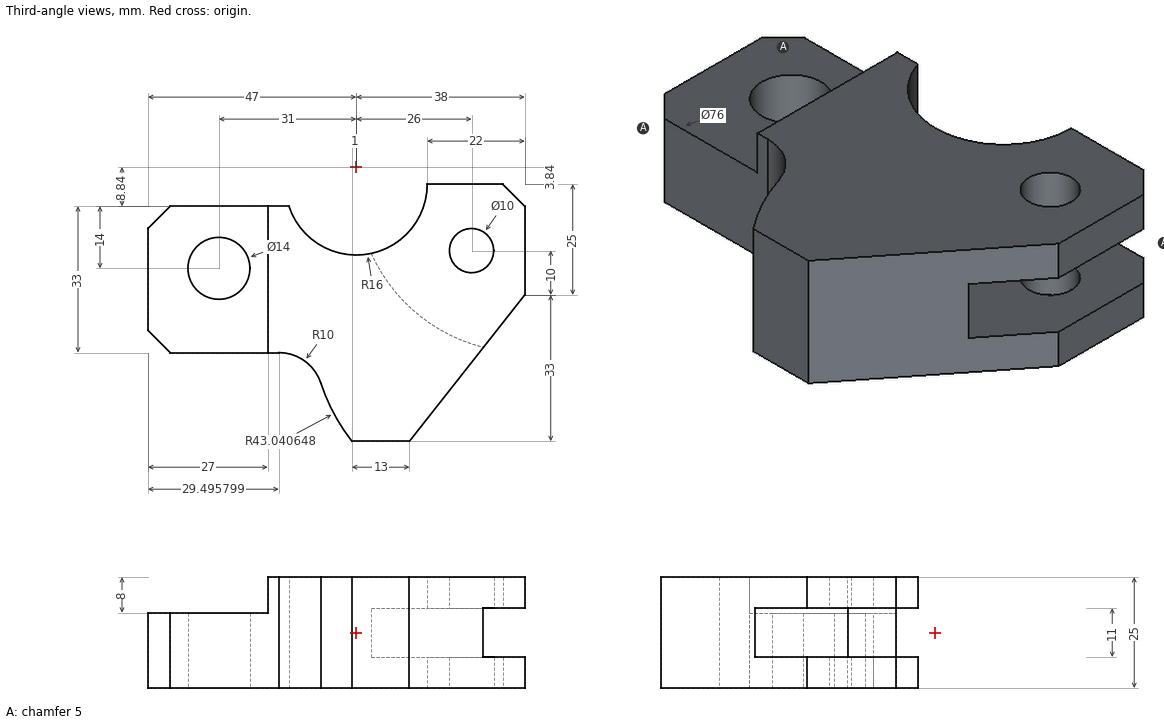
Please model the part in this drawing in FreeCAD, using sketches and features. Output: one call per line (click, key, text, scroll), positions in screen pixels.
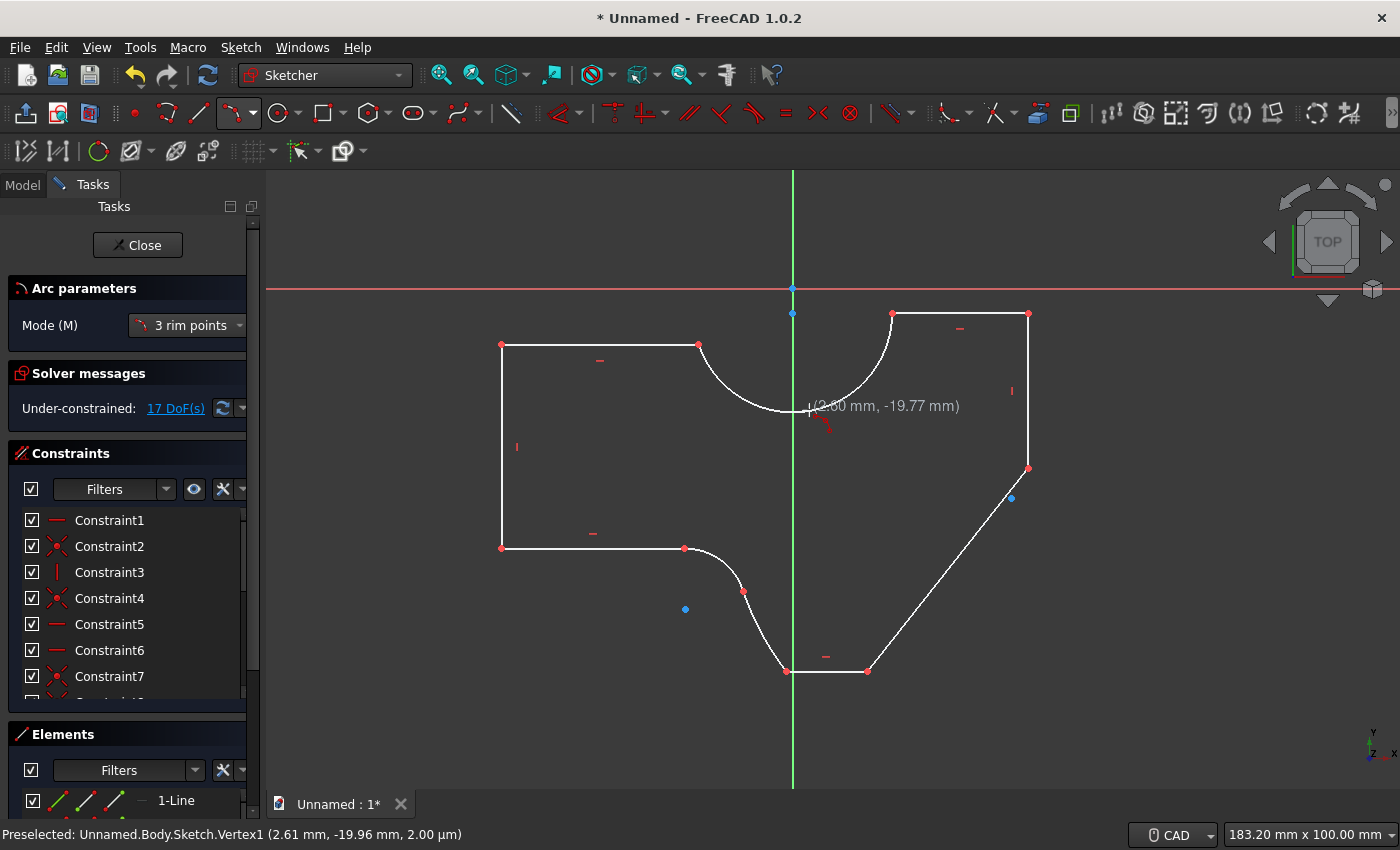
key(g)
key(c)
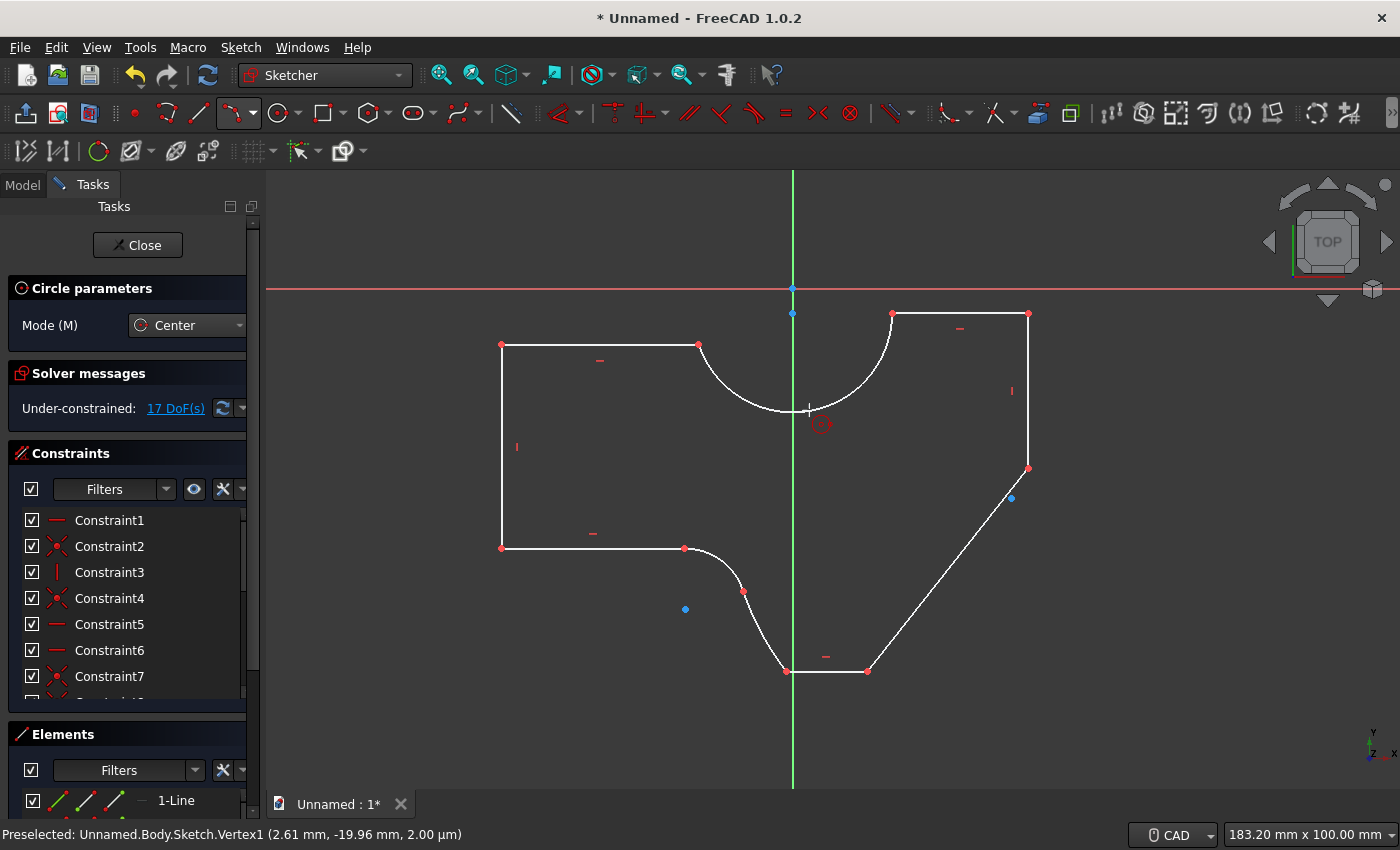
click(601, 430)
move(632, 399)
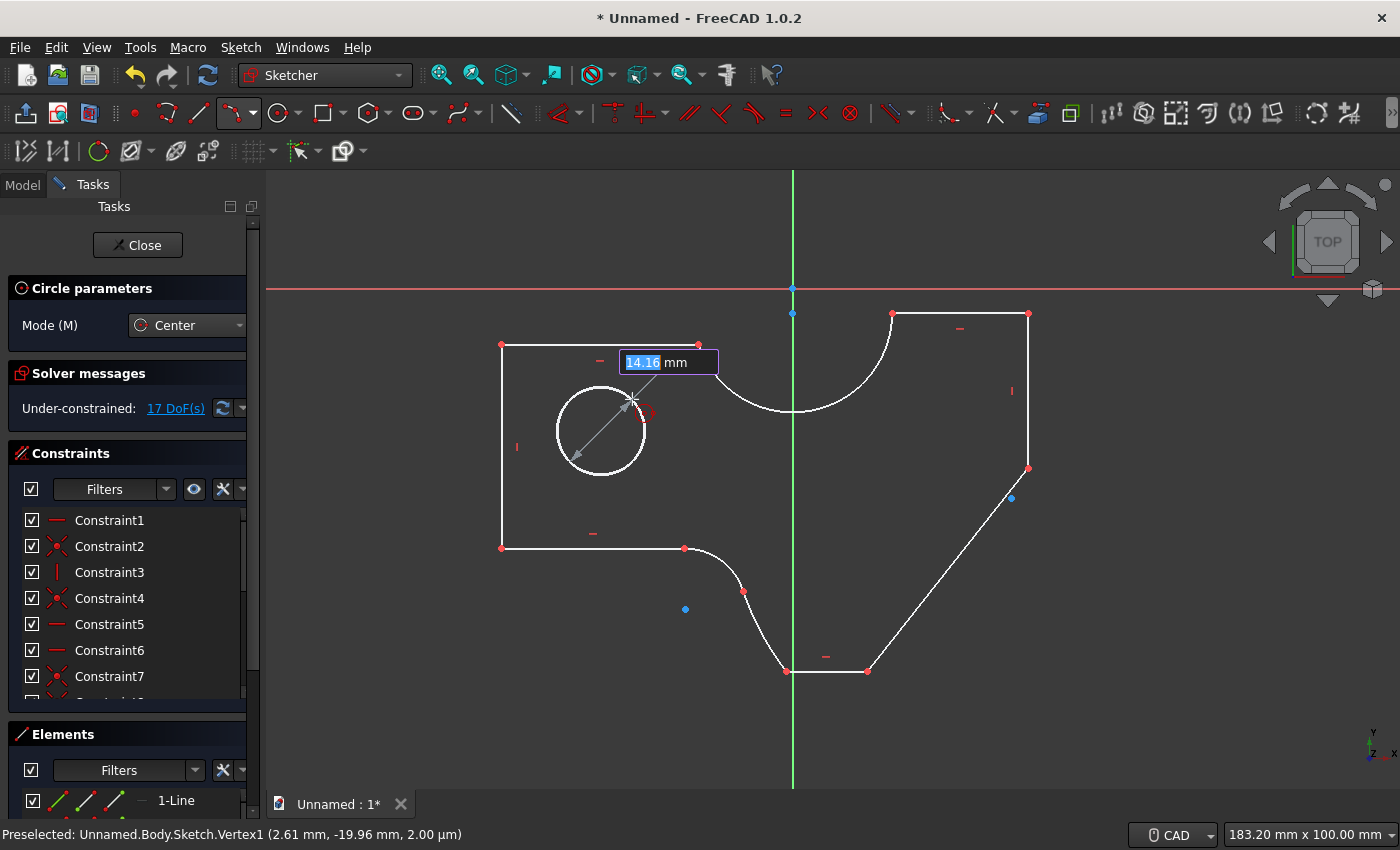
text(14)
key(Return)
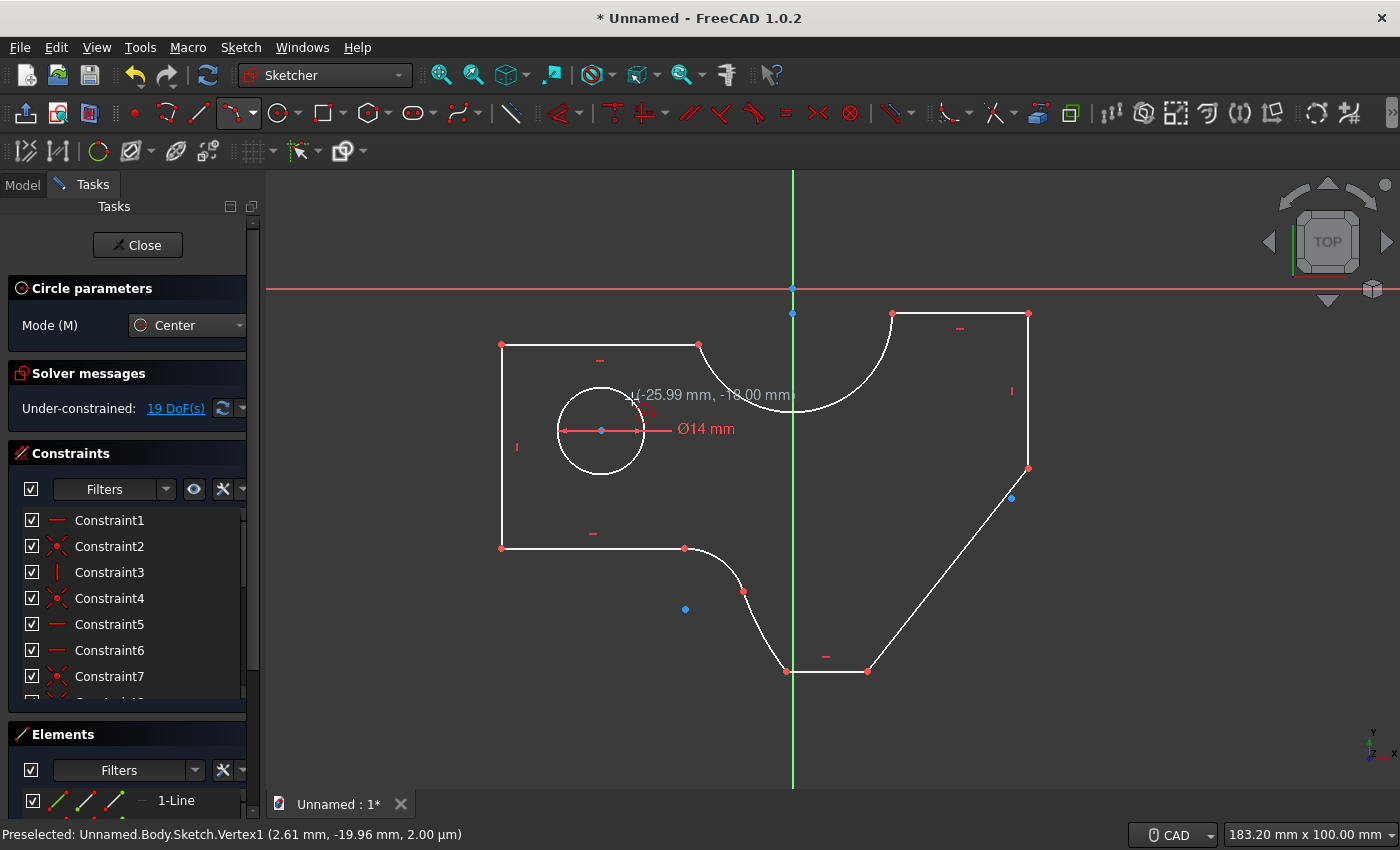
click(954, 405)
move(976, 383)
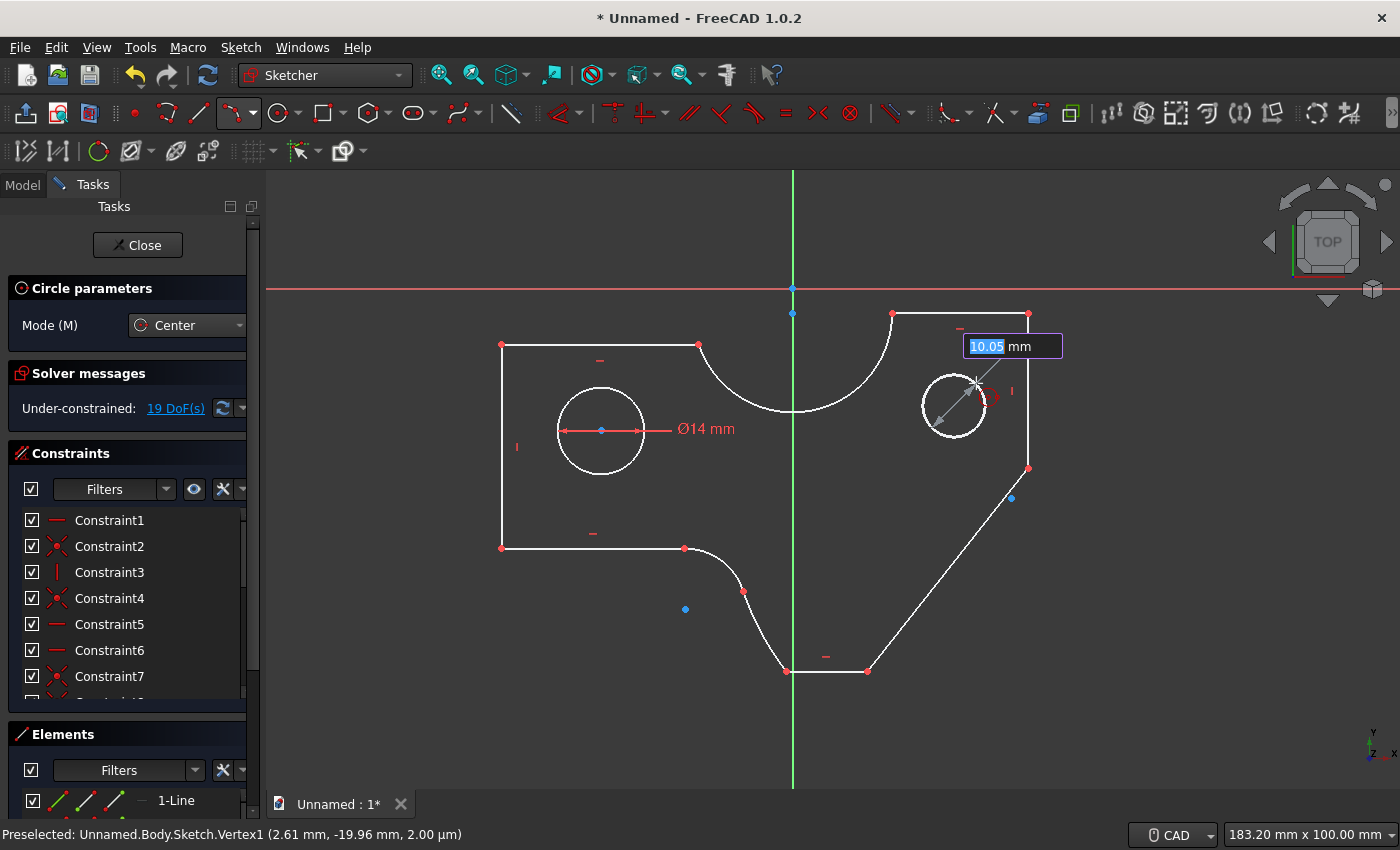
text(10)
key(Return)
key(Escape)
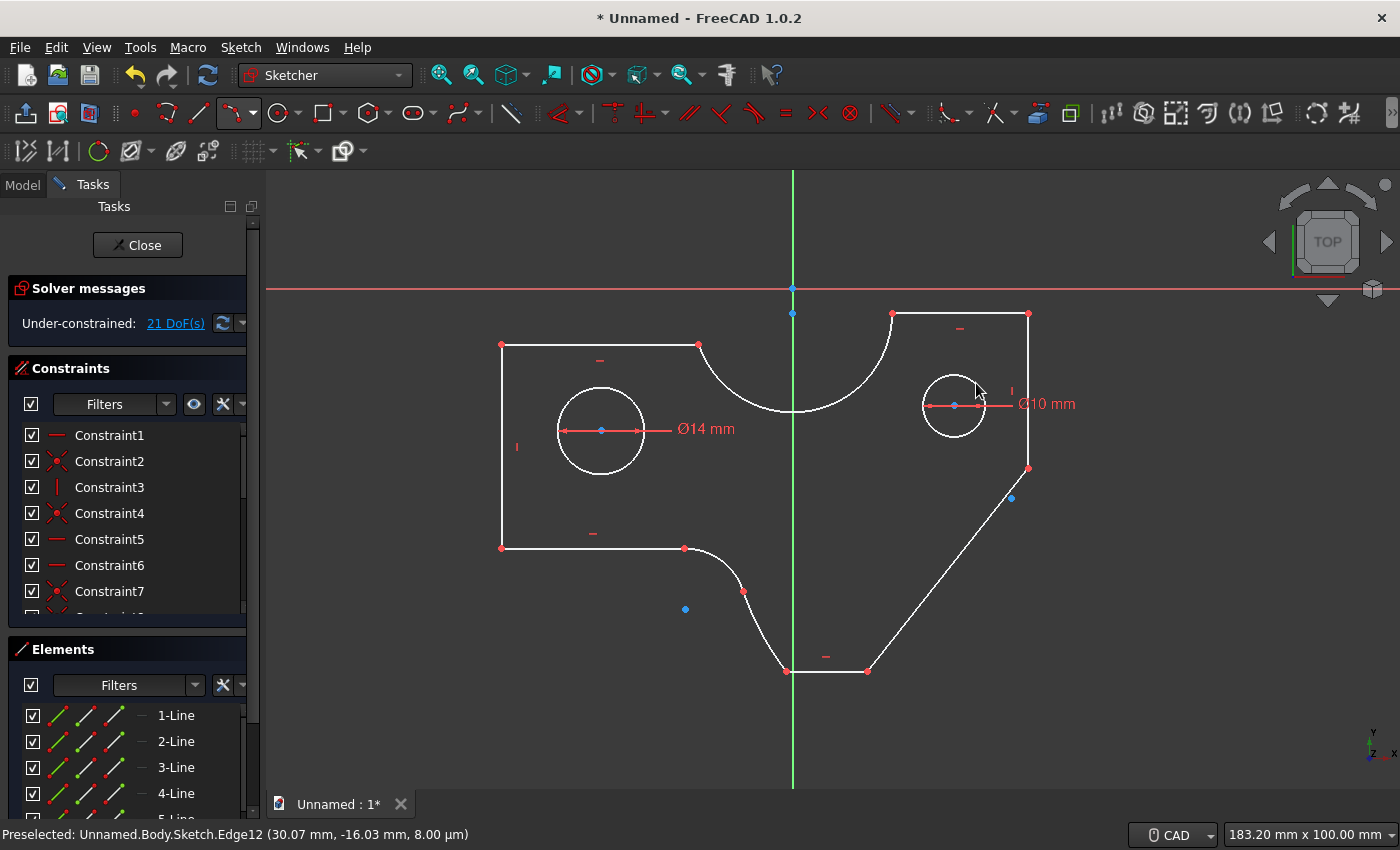
click(557, 549)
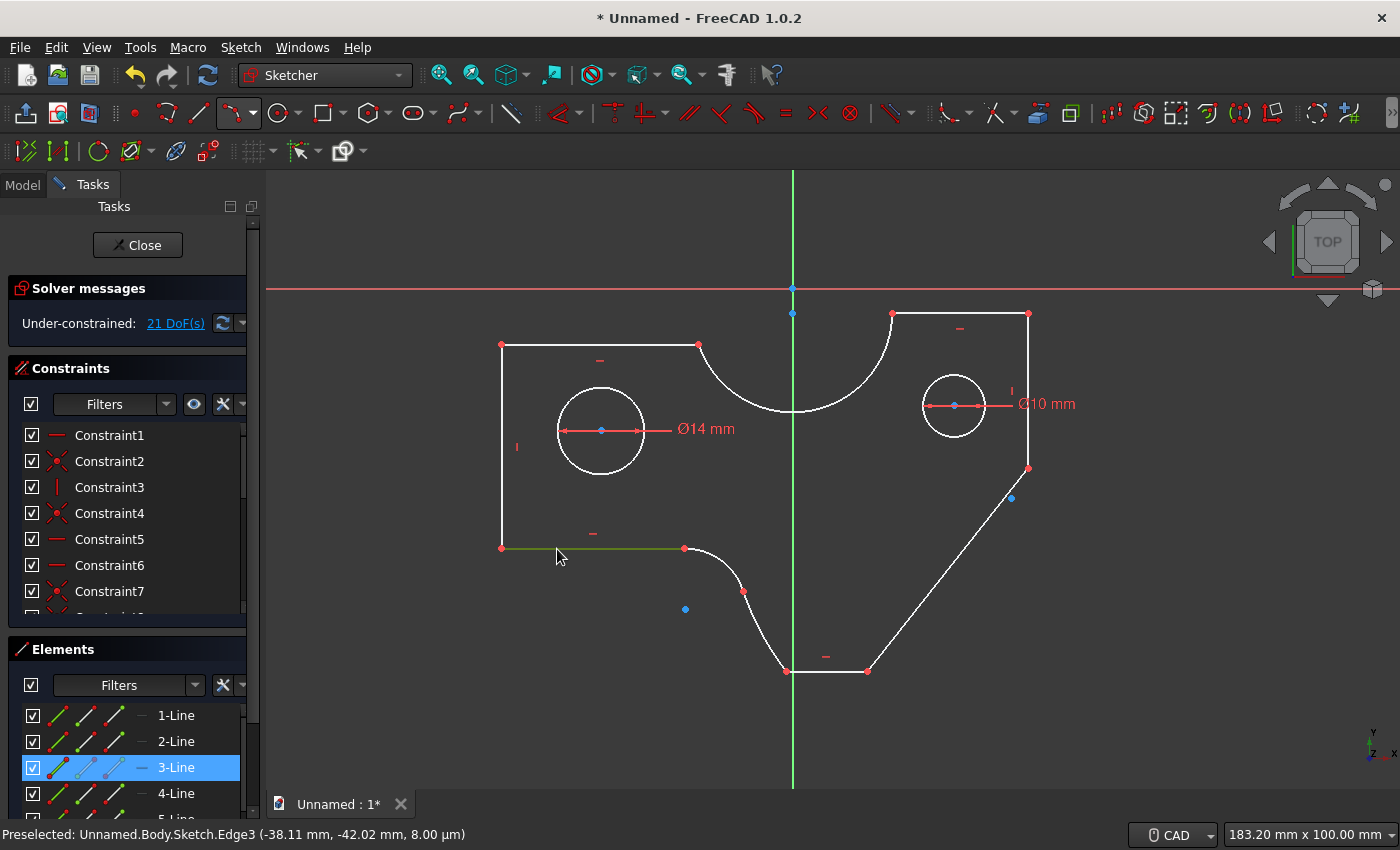
click(732, 571)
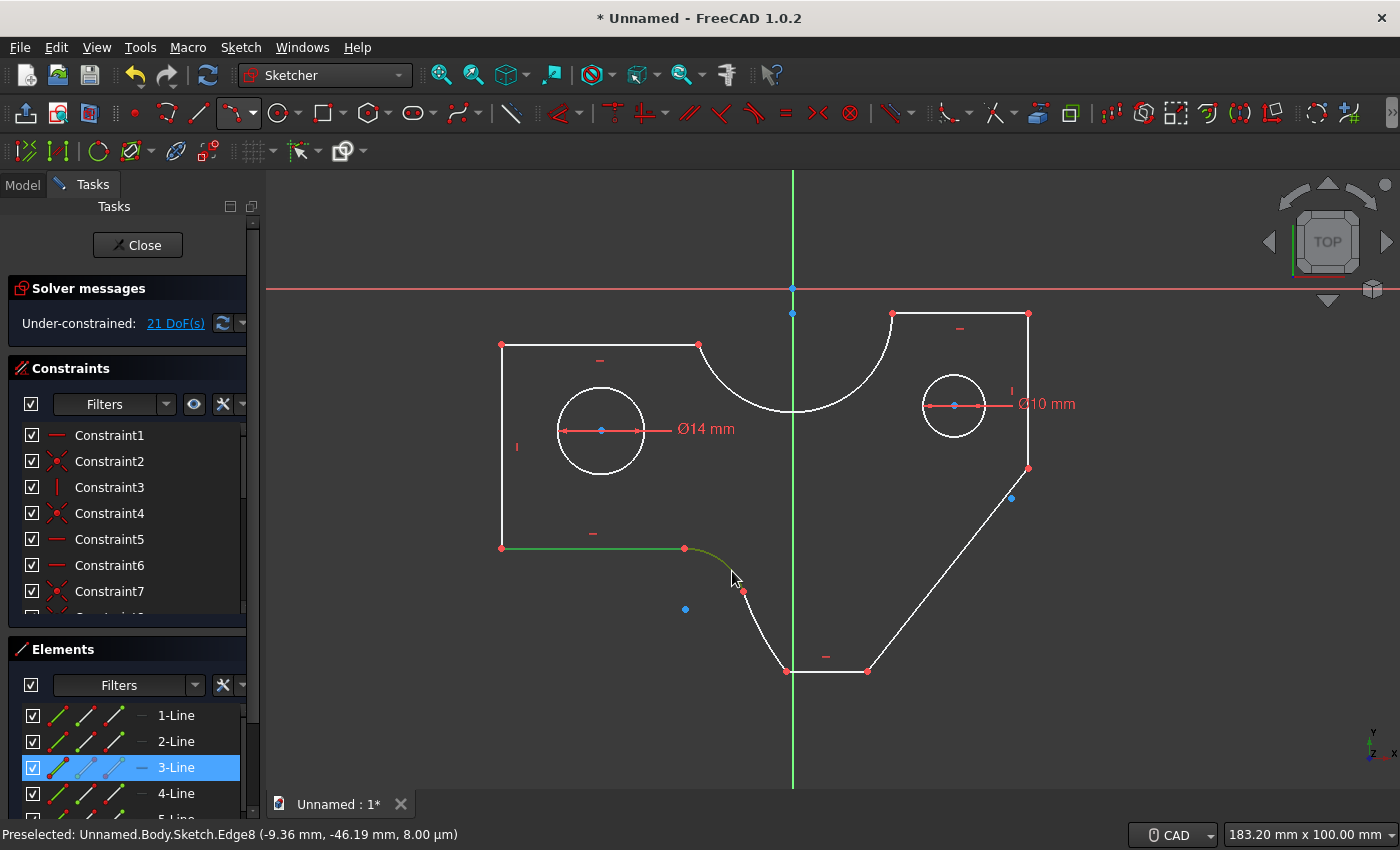
key(t)